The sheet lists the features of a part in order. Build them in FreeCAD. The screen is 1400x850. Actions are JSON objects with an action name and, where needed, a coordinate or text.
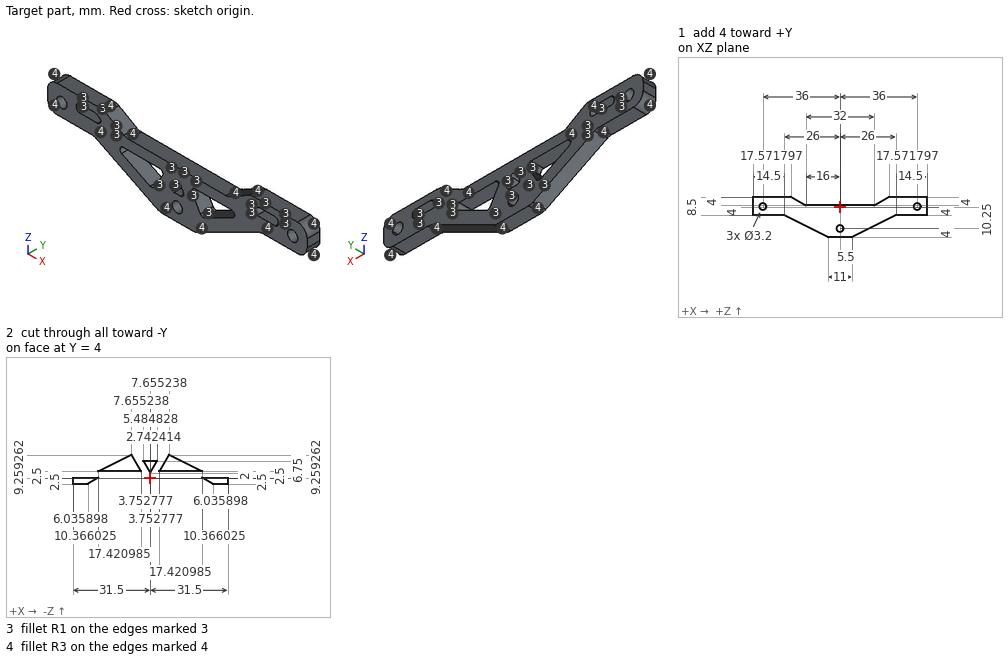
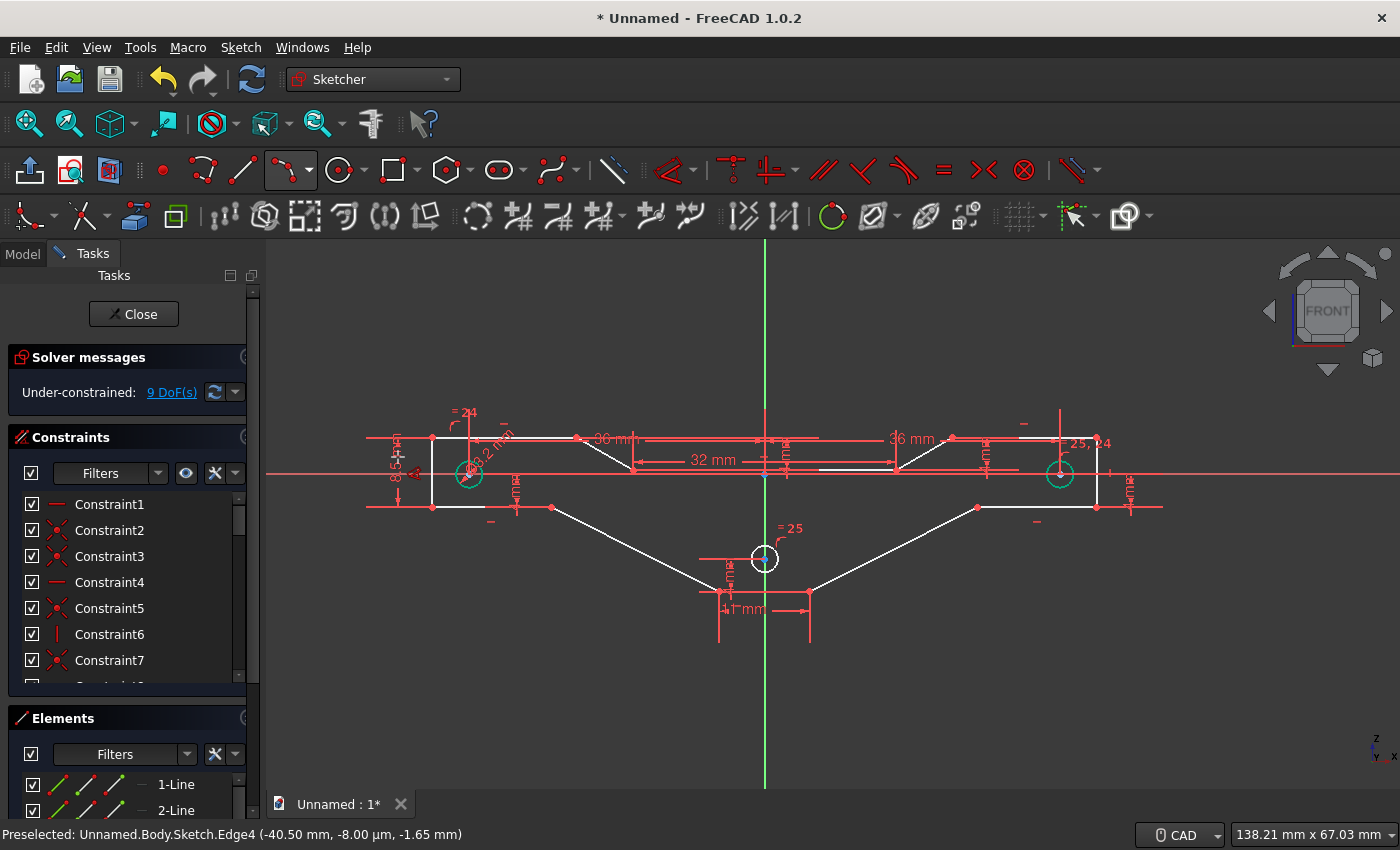
{"action": "left_click", "coordinate": [551, 507]}
{"action": "left_click", "coordinate": [707, 440]}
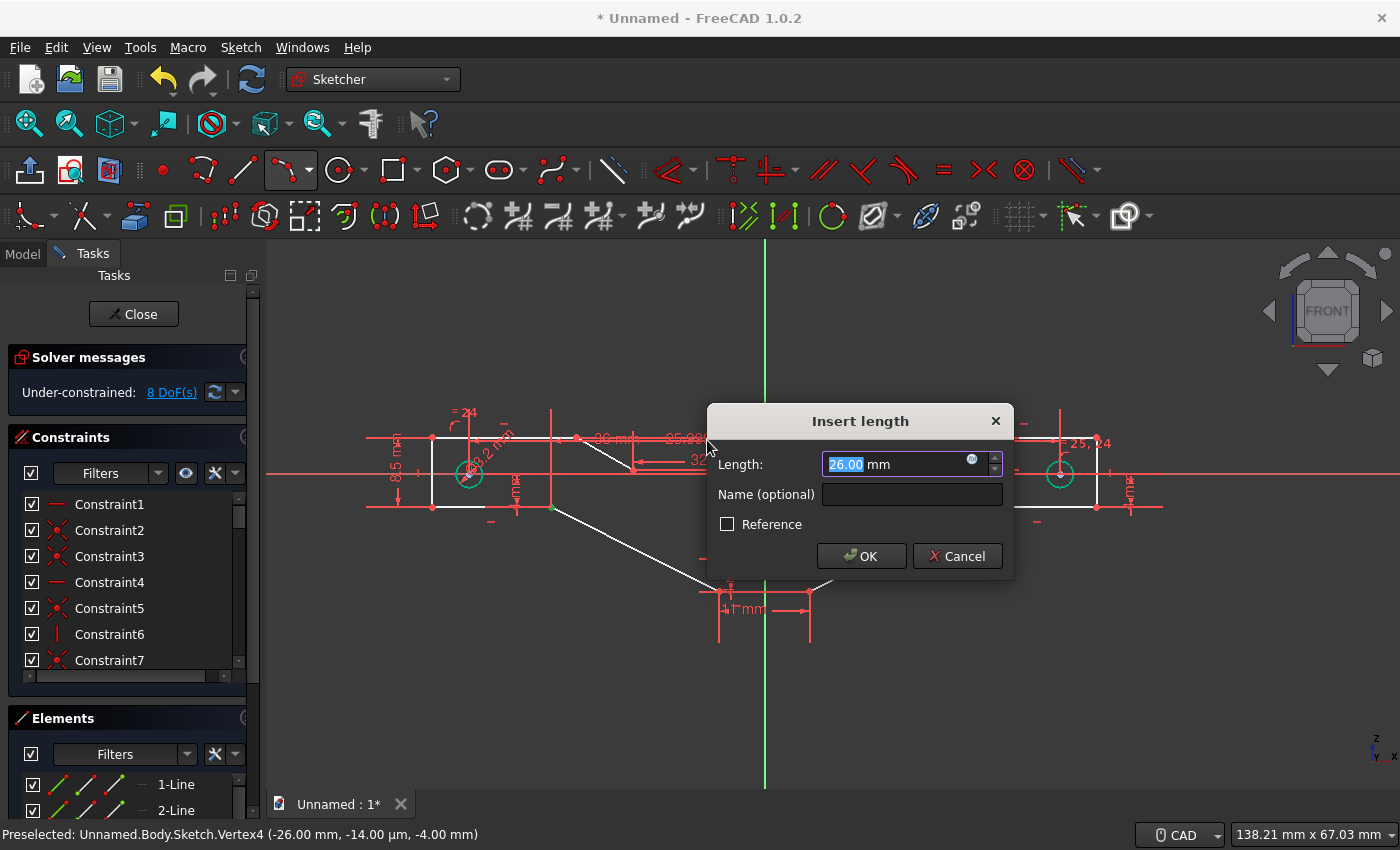
{"action": "type", "text": "26"}
{"action": "key", "text": "Return"}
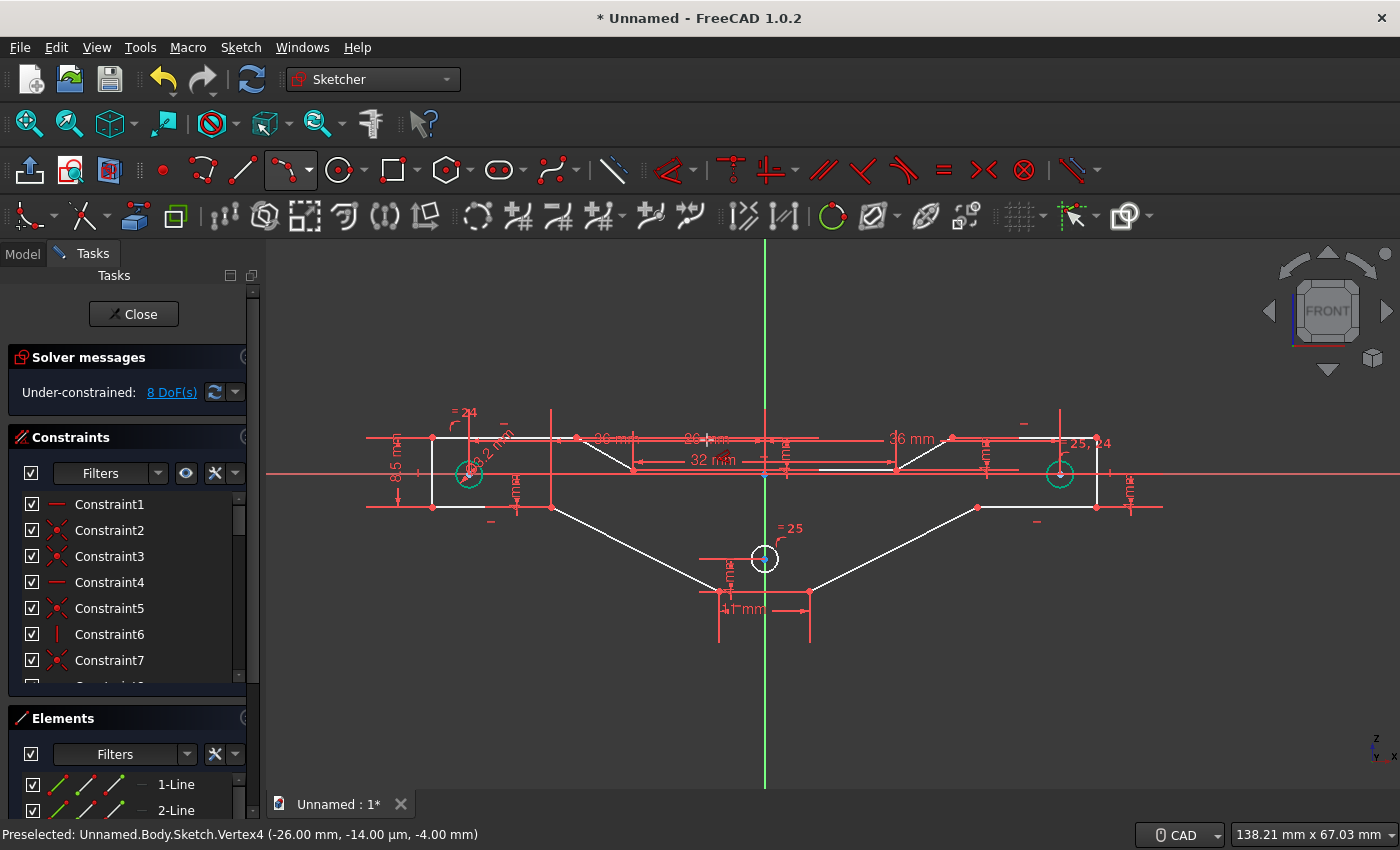
{"action": "left_click", "coordinate": [633, 470]}
{"action": "left_click", "coordinate": [699, 508]}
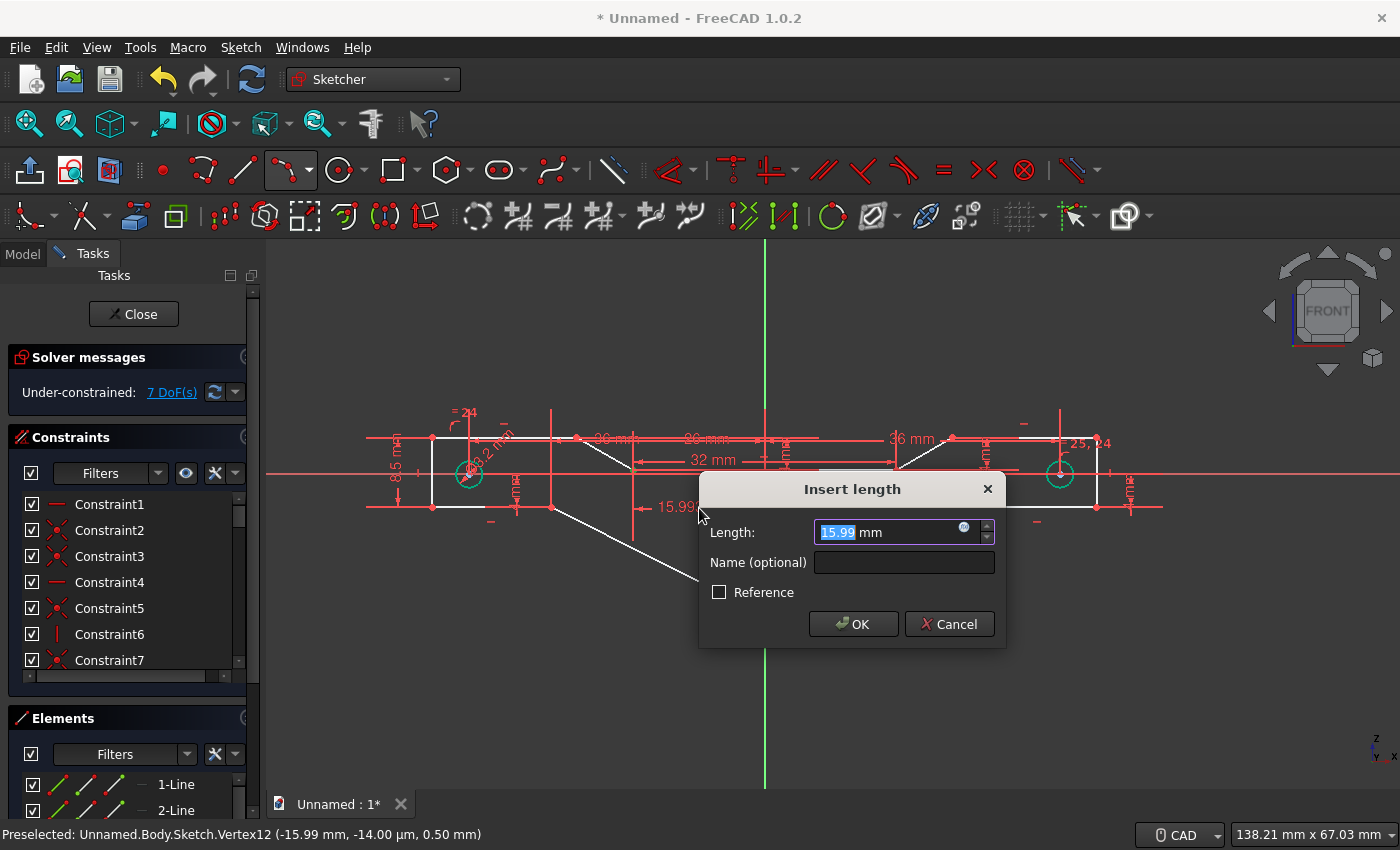
{"action": "type", "text": "16"}
{"action": "key", "text": "Return"}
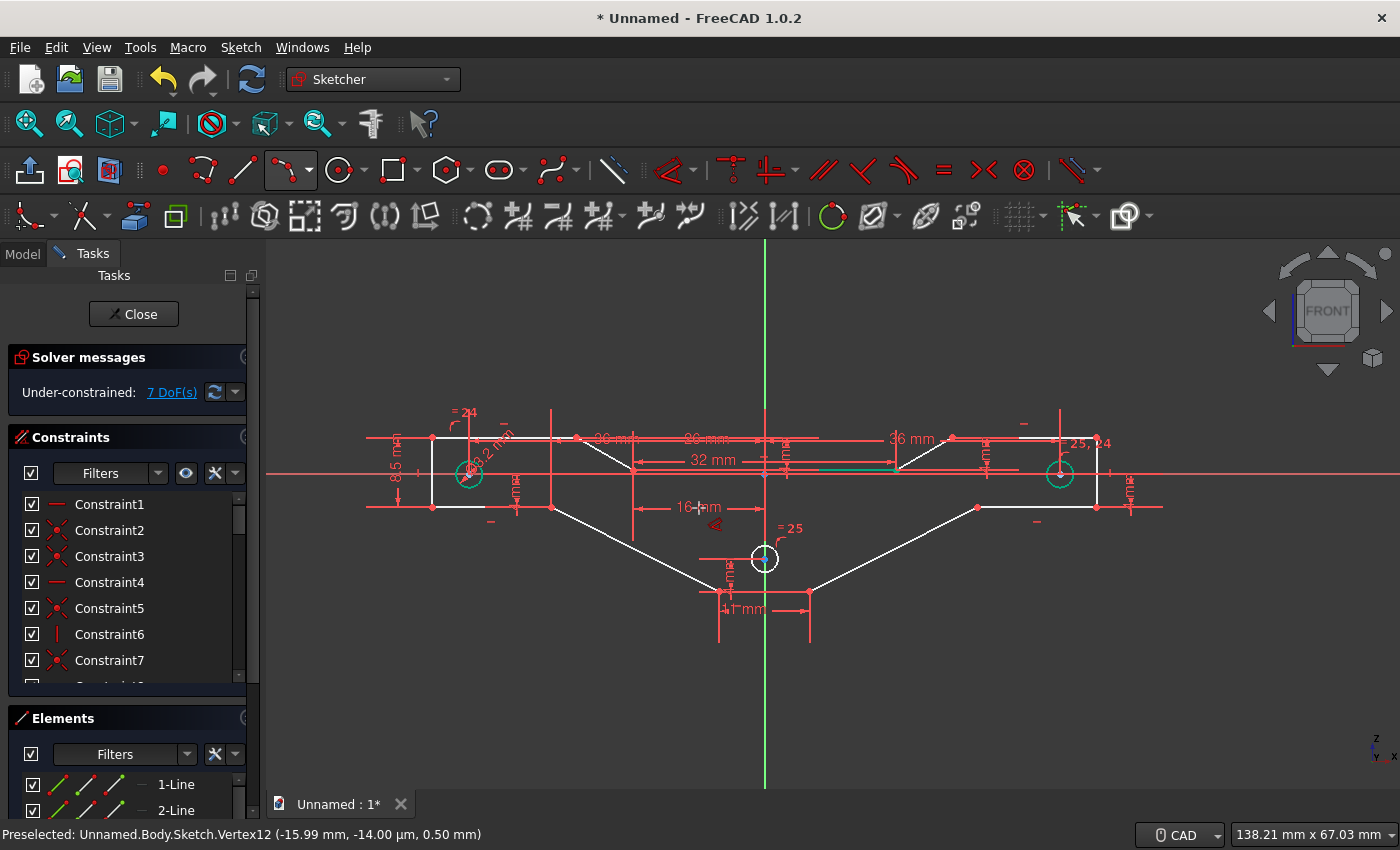
{"action": "left_click", "coordinate": [978, 507]}
{"action": "left_click", "coordinate": [871, 541]}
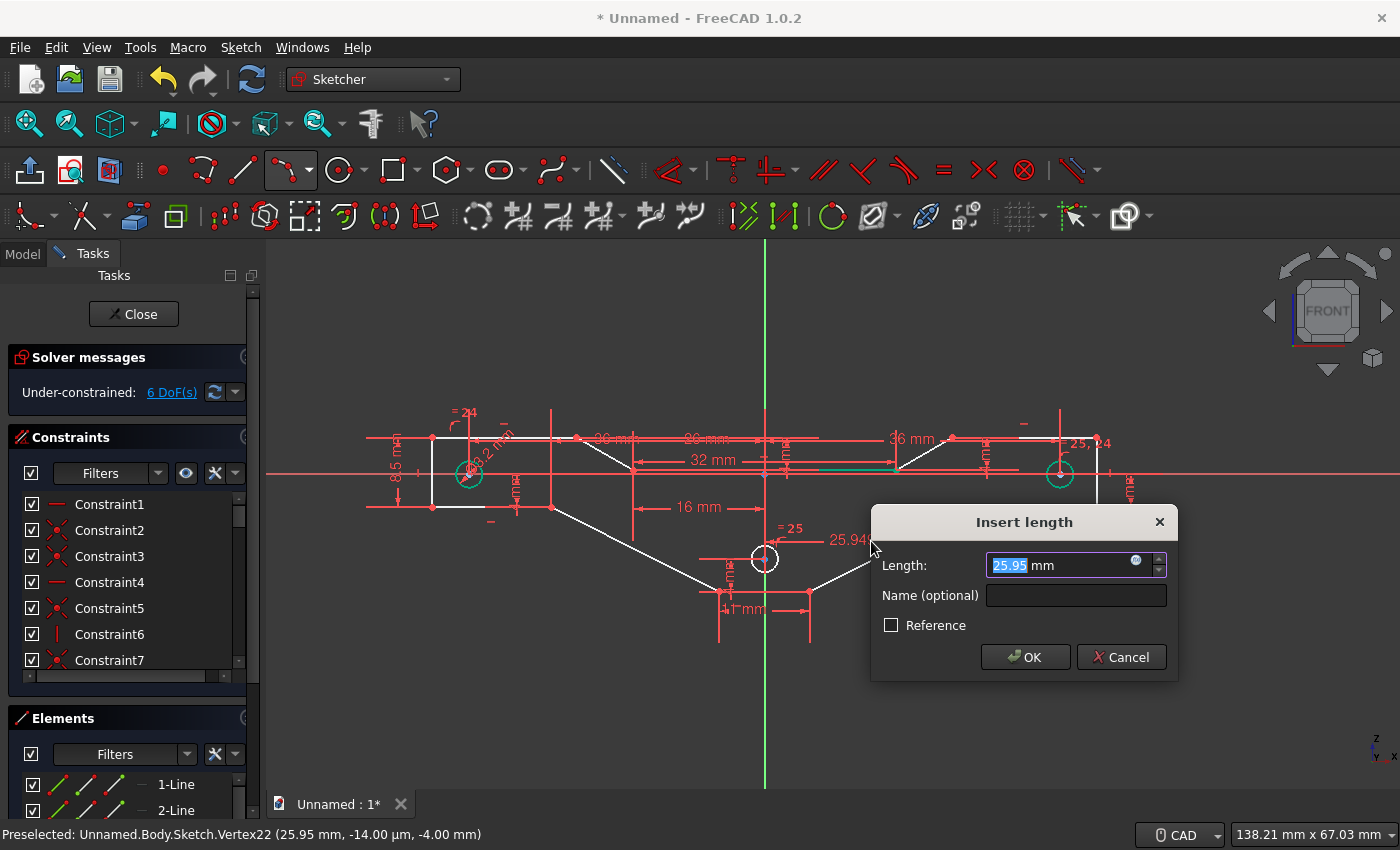
{"action": "type", "text": "26"}
{"action": "key", "text": "Return"}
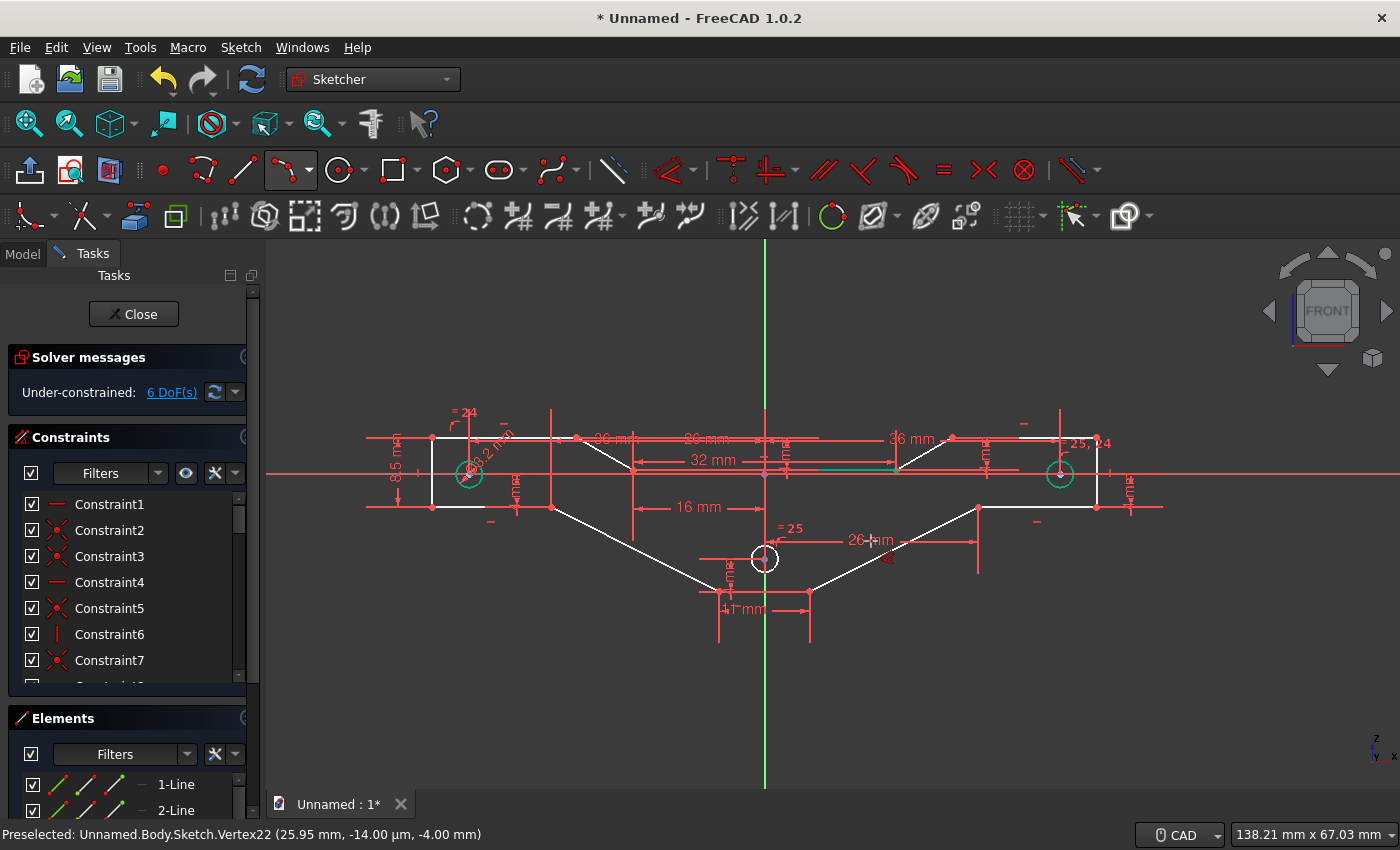
{"action": "left_click", "coordinate": [516, 507]}
{"action": "left_click", "coordinate": [492, 541]}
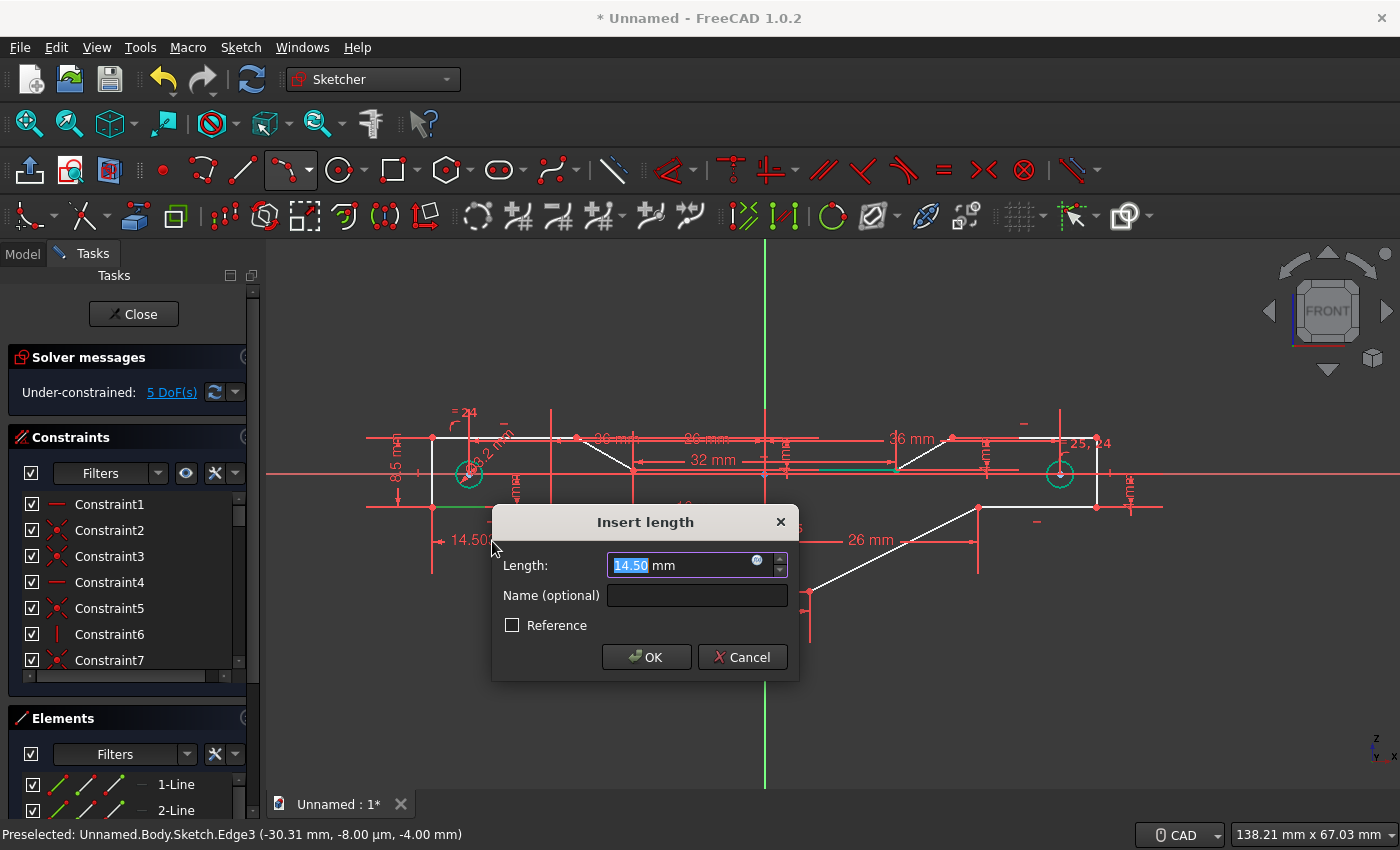
{"action": "type", "text": "14.5"}
{"action": "key", "text": "Return"}